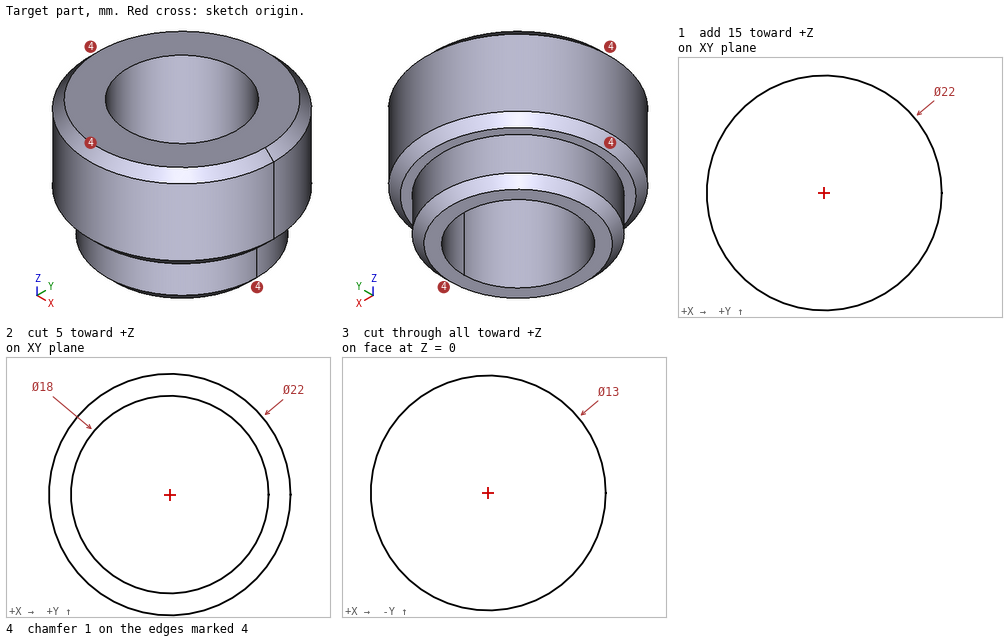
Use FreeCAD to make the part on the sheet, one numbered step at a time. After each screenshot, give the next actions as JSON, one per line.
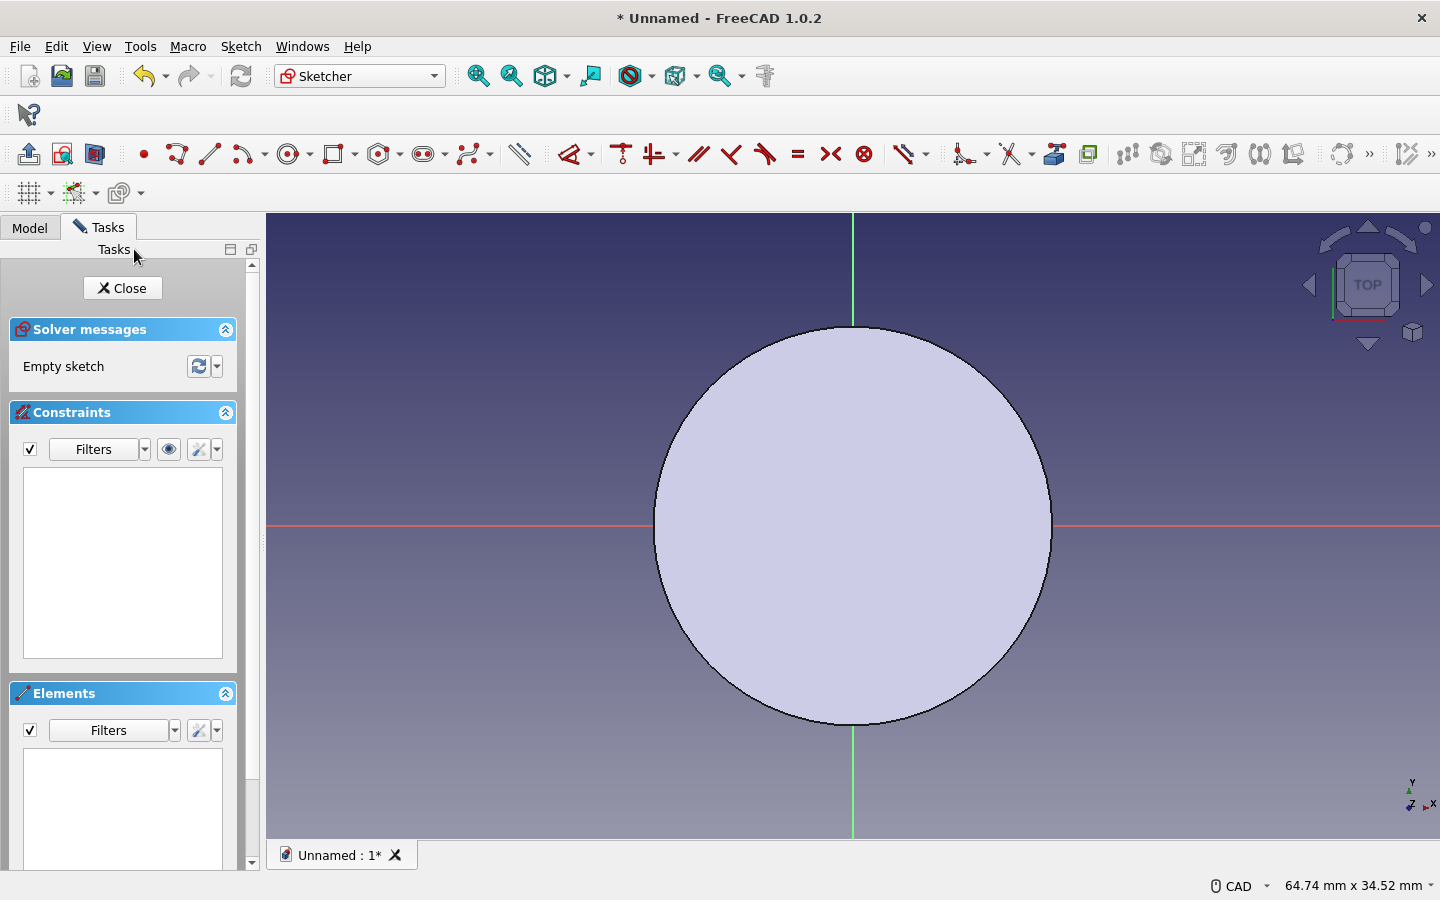
{"action": "key", "text": "q s"}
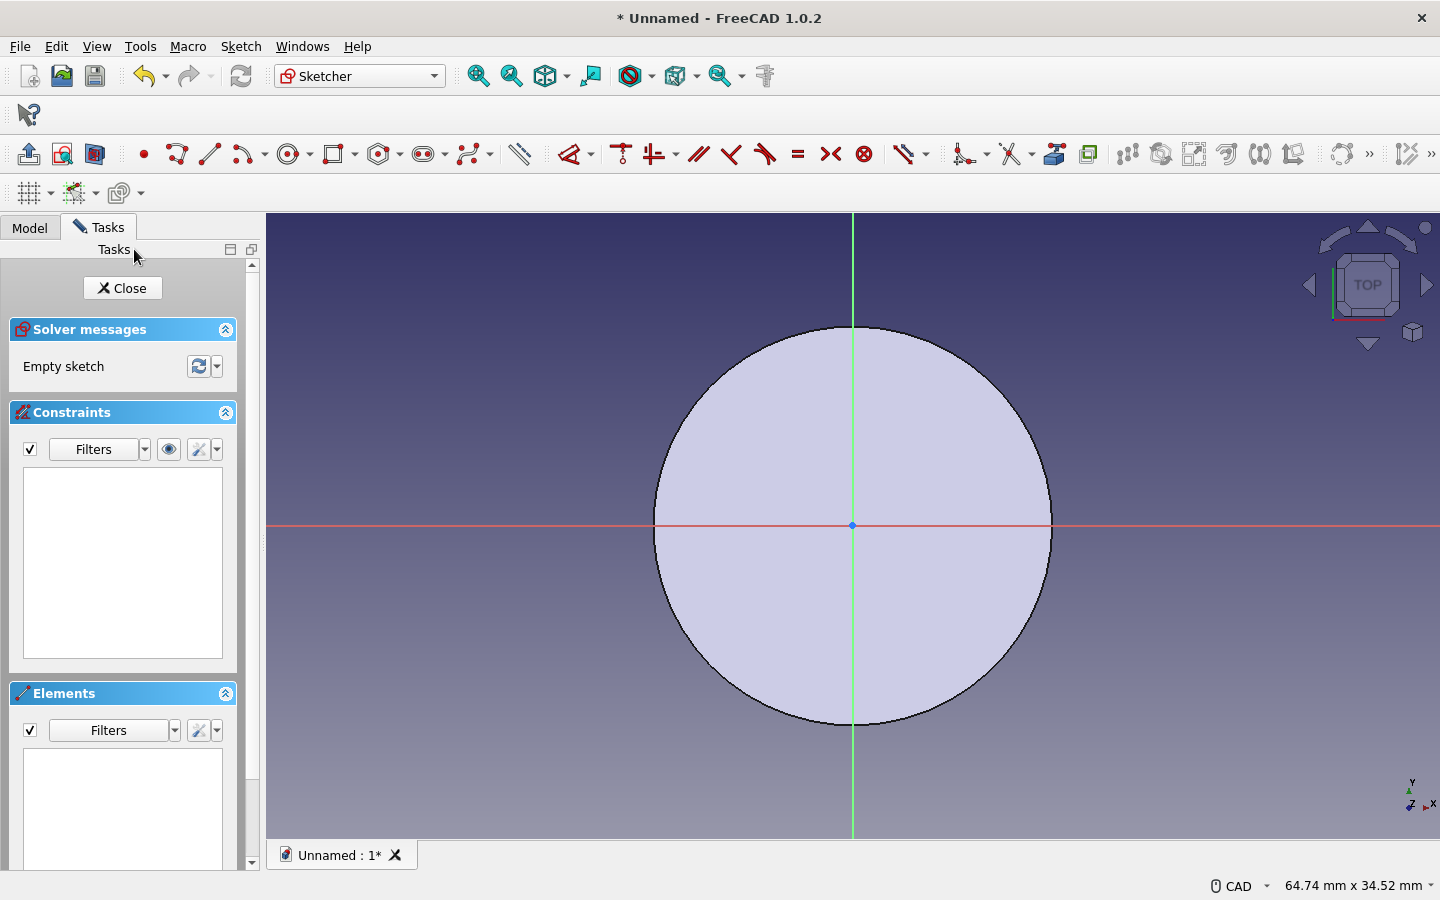
{"action": "left_click", "coordinate": [288, 154]}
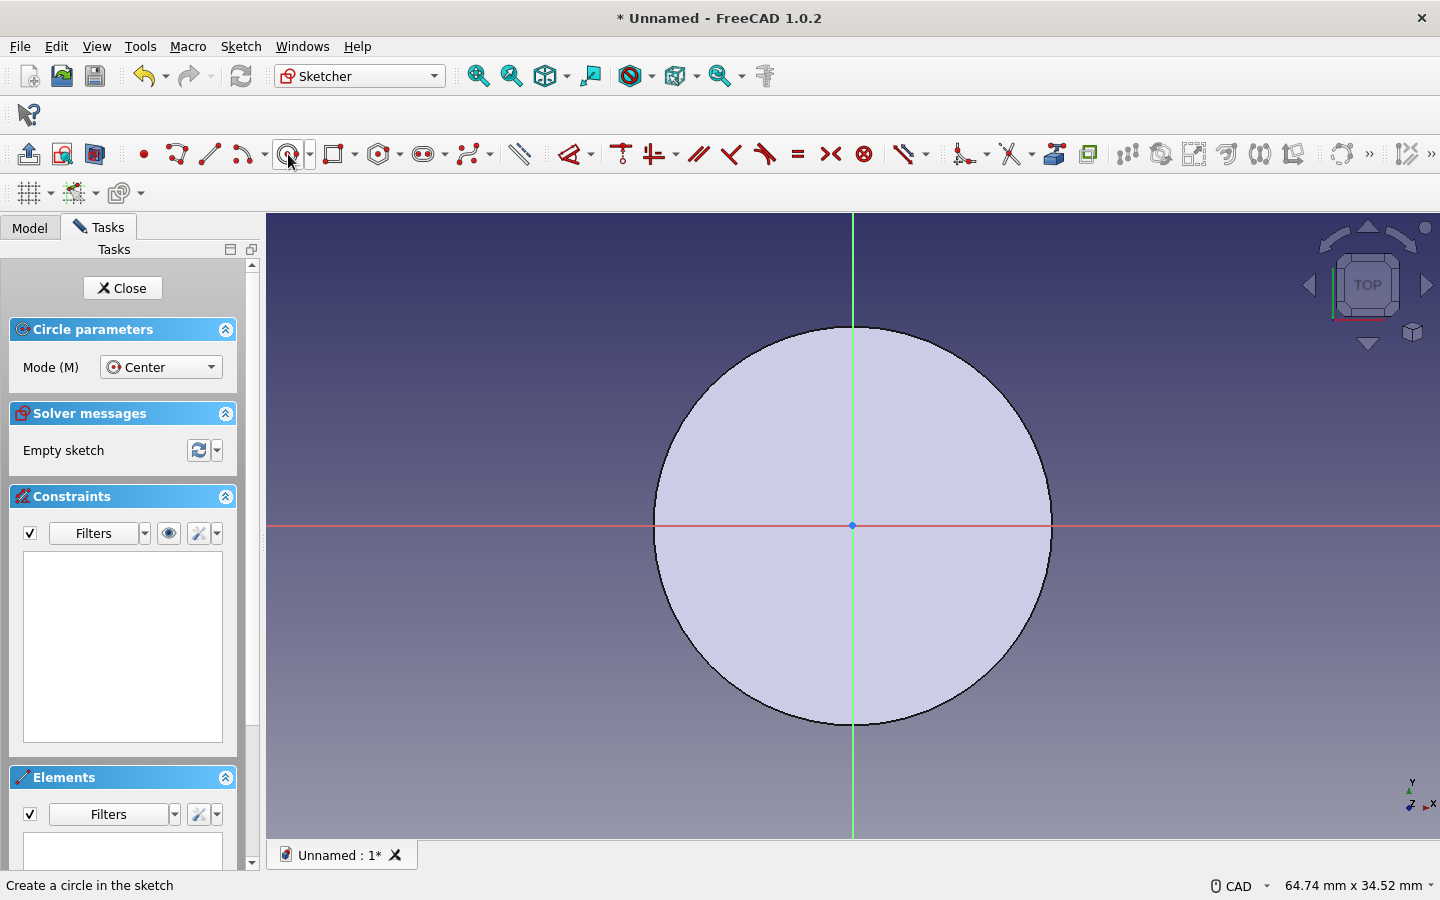
{"action": "left_click", "coordinate": [853, 526]}
{"action": "mouse_move", "coordinate": [994, 385]}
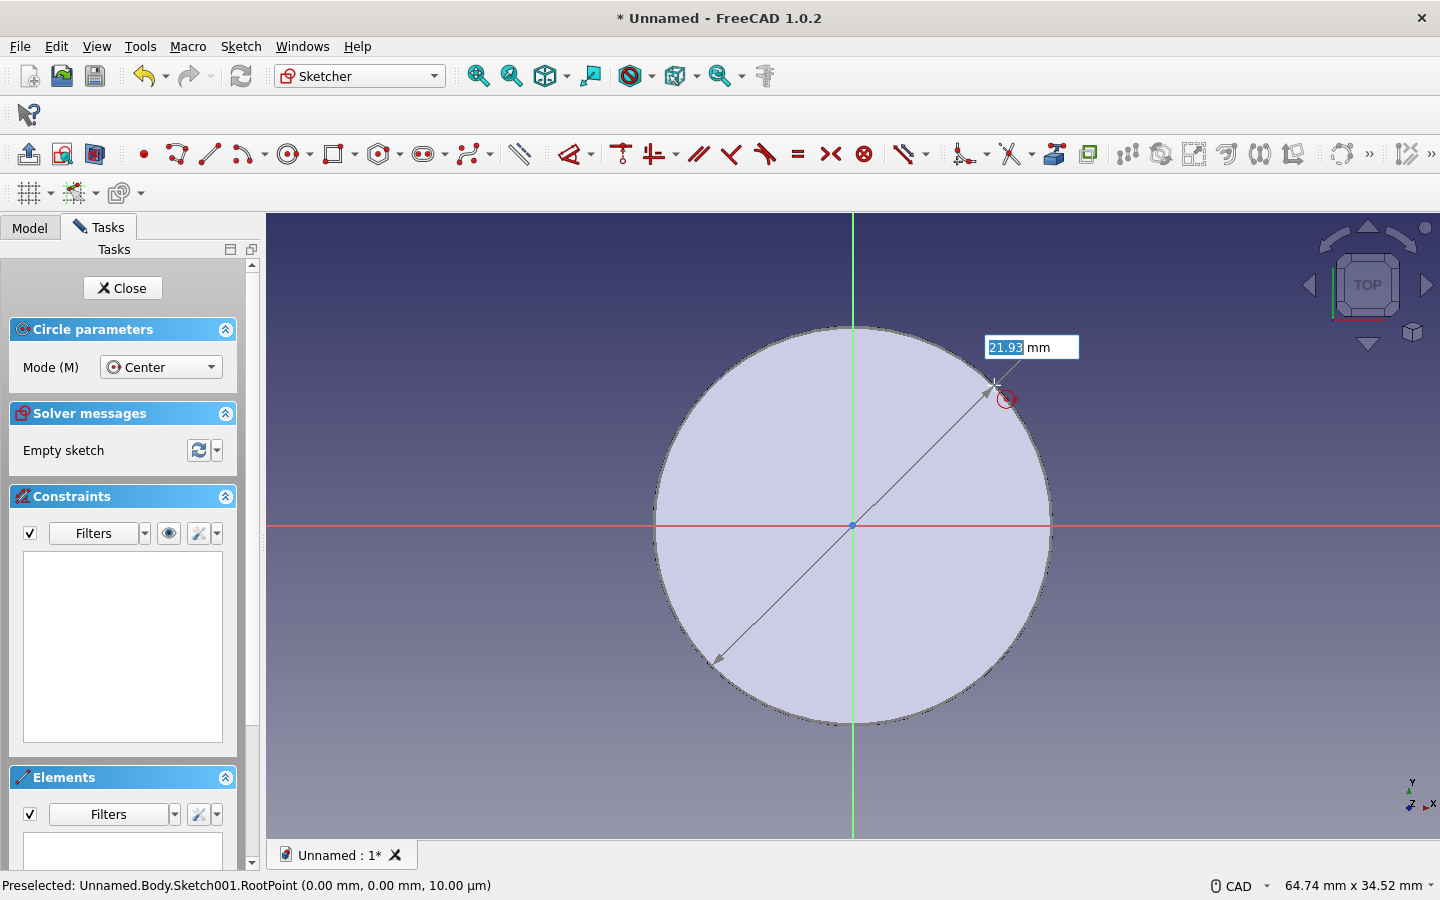
{"action": "type", "text": "22"}
{"action": "key", "text": "Return"}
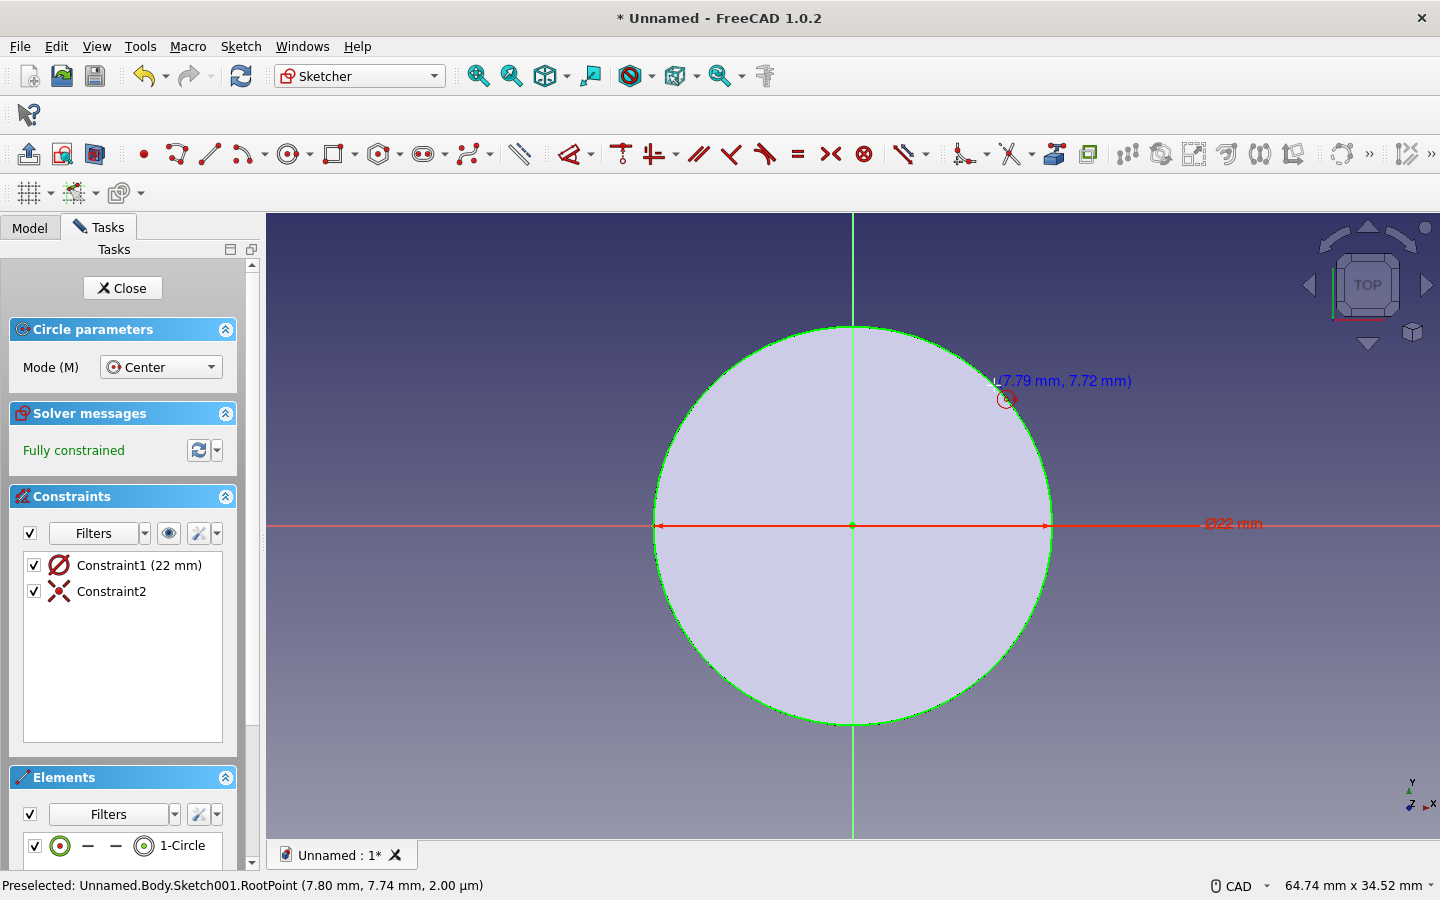
{"action": "left_click", "coordinate": [853, 526]}
{"action": "mouse_move", "coordinate": [968, 411]}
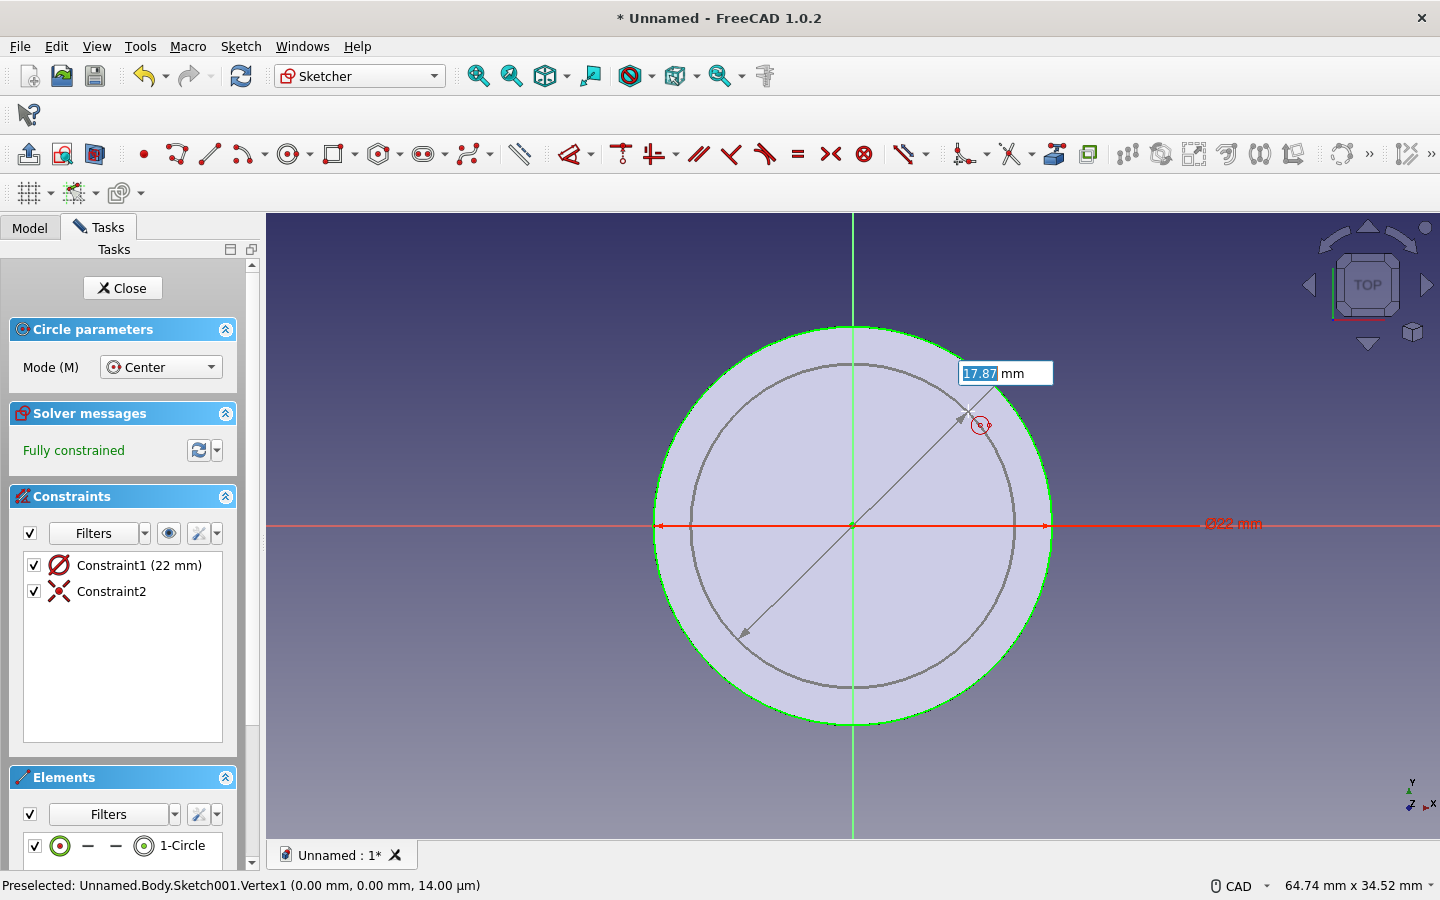
{"action": "type", "text": "18"}
{"action": "key", "text": "Return"}
{"action": "key", "text": "Escape"}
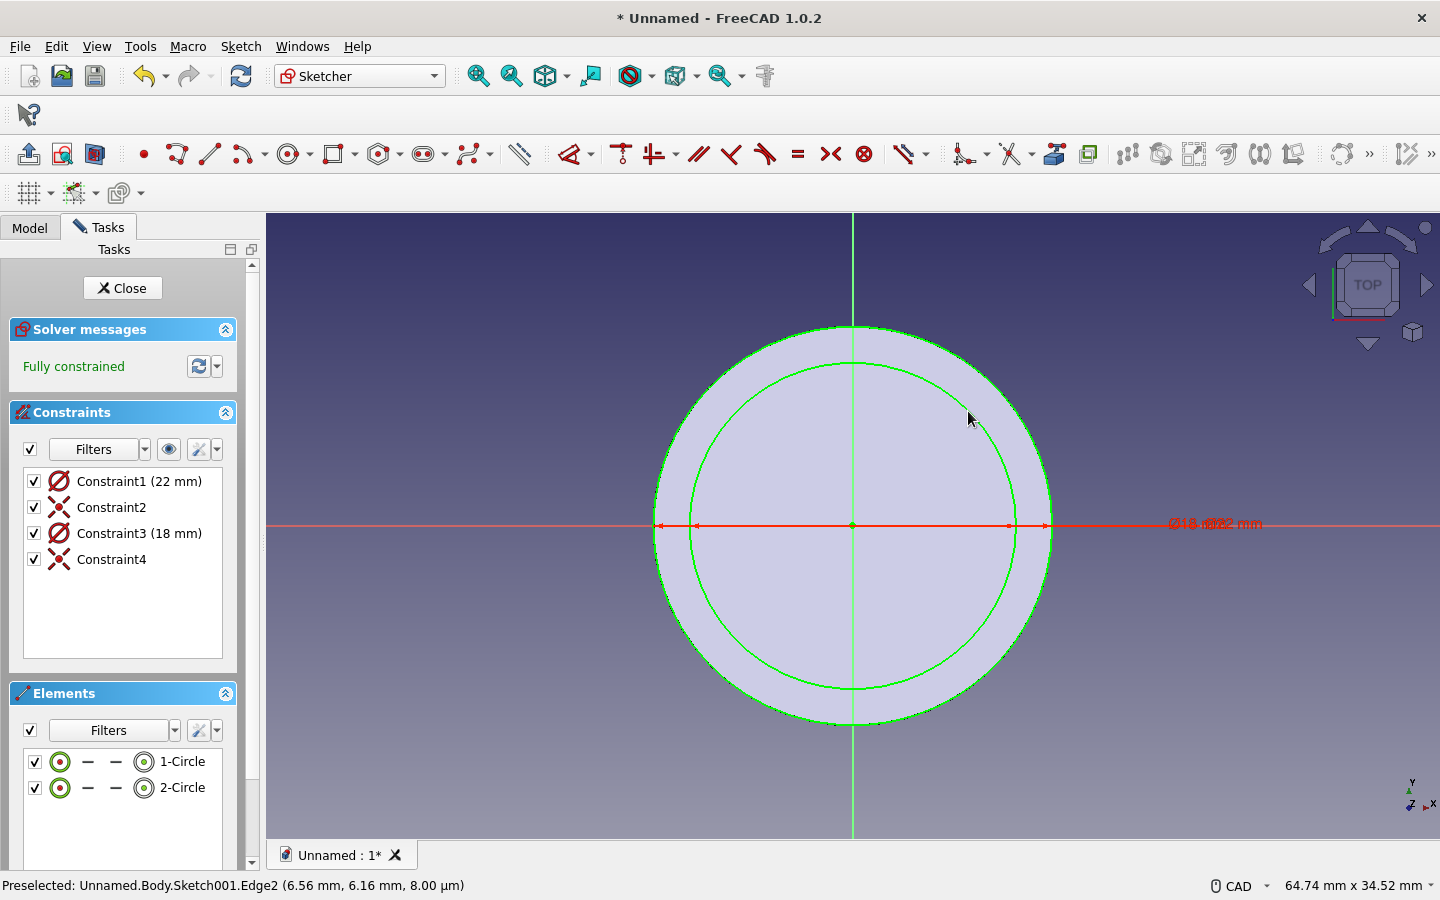
{"action": "left_click", "coordinate": [123, 288]}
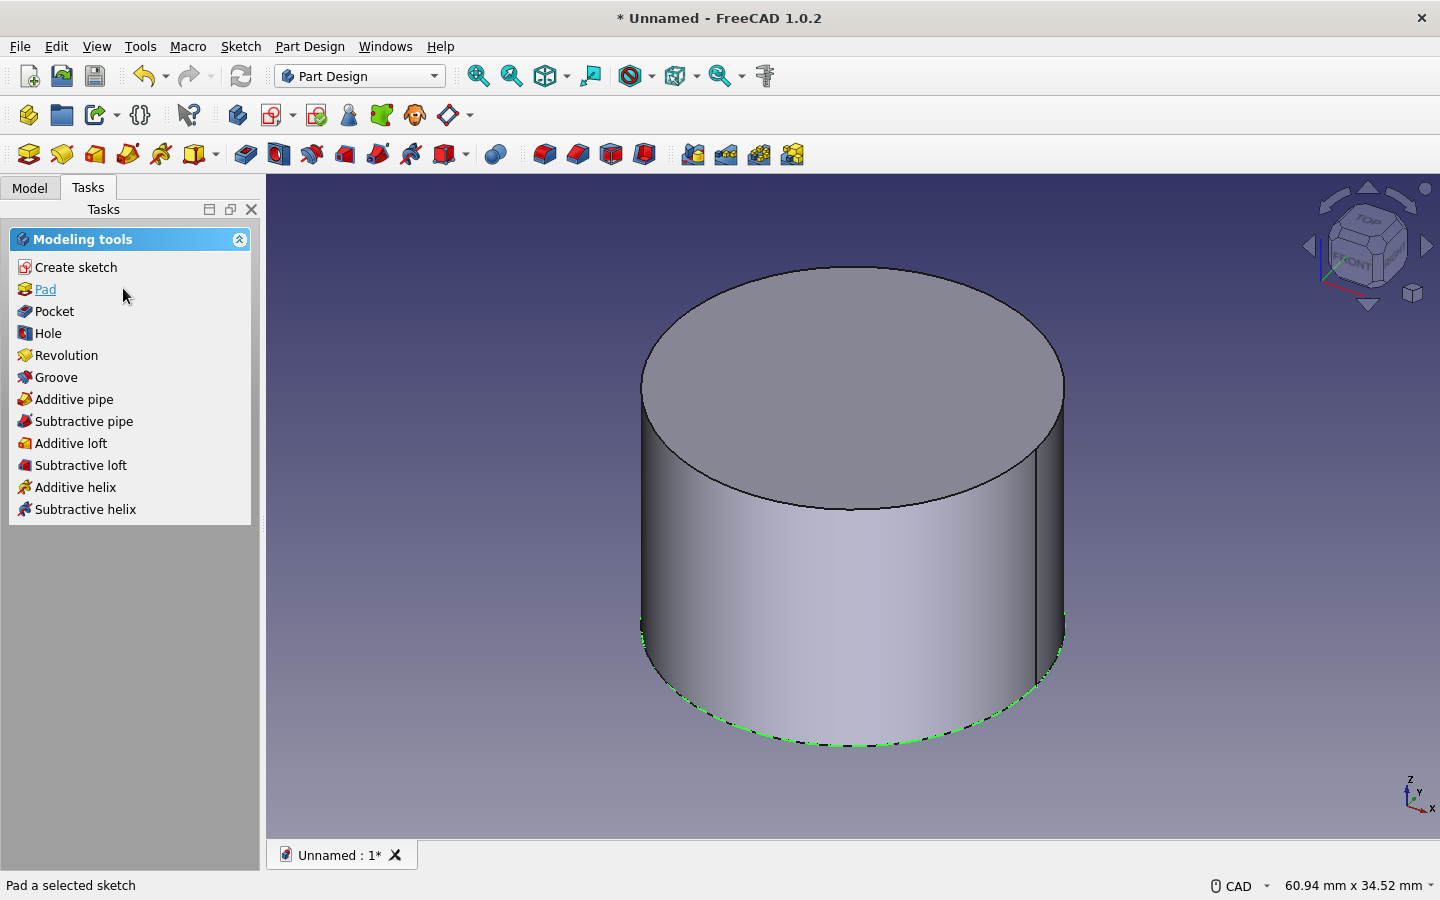
{"action": "left_click", "coordinate": [246, 154]}